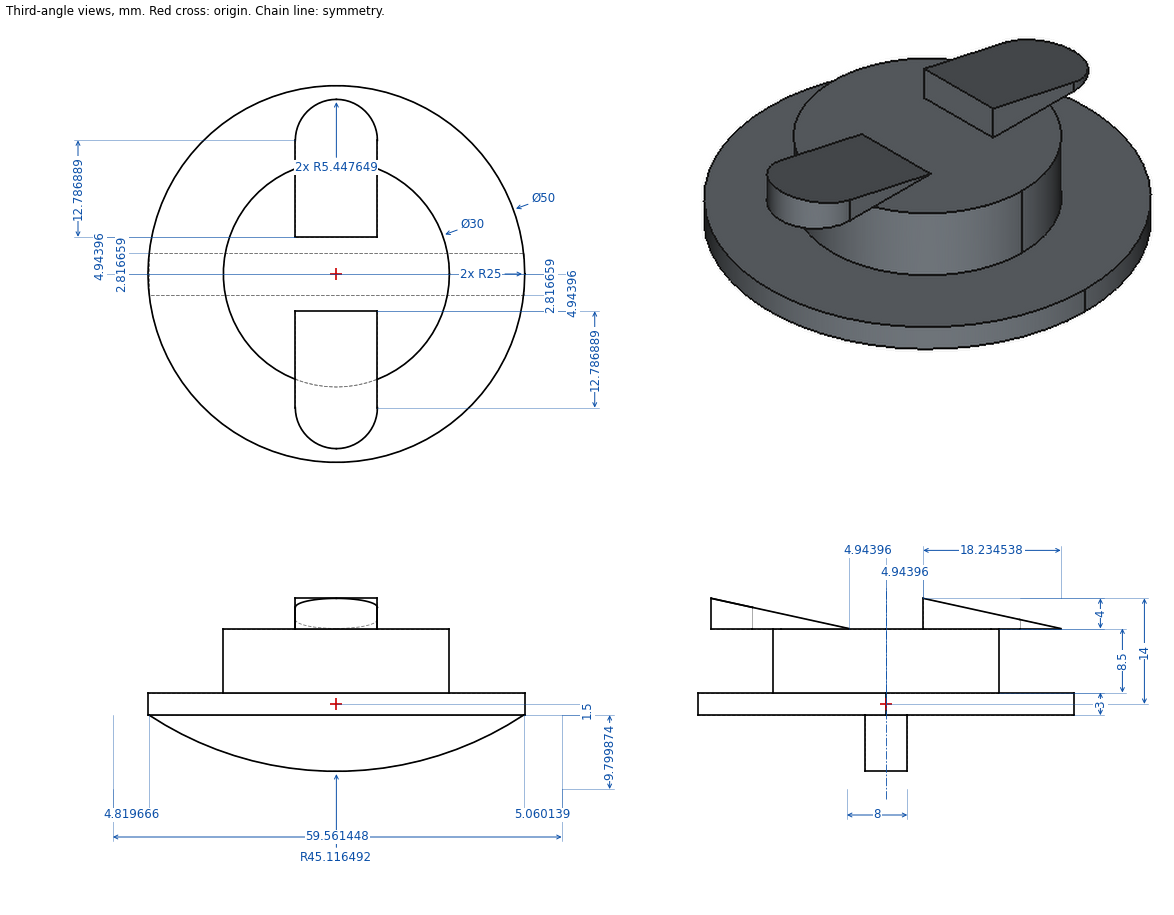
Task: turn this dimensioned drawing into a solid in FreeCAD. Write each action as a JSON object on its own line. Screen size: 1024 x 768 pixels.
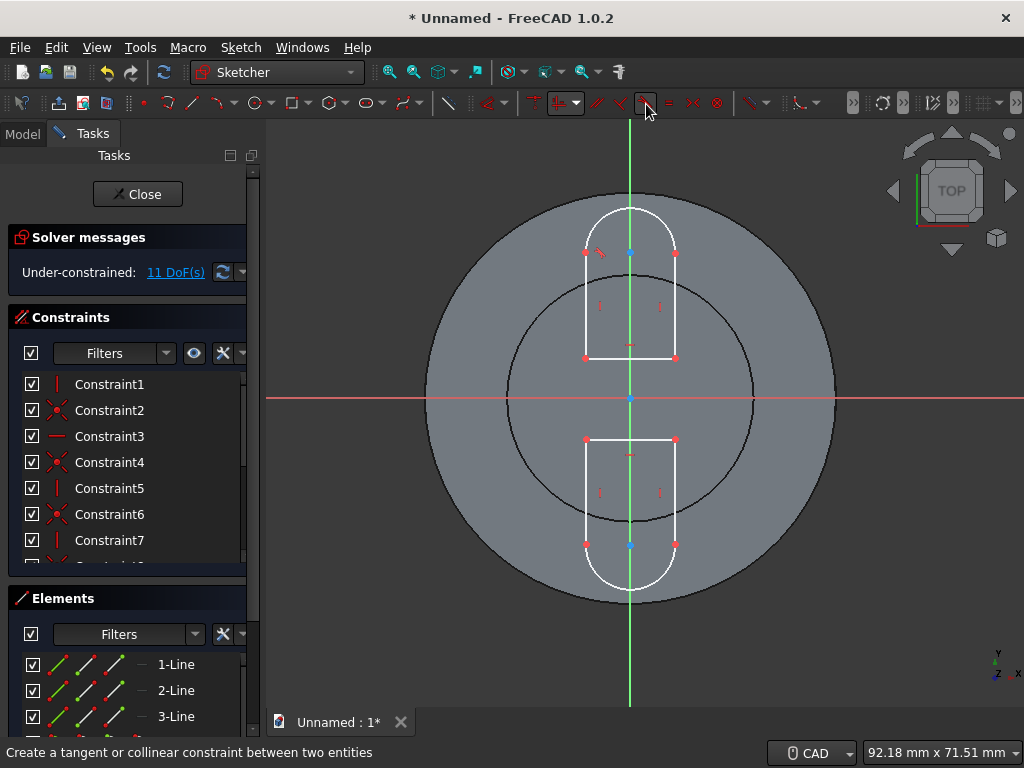
{"action": "left_click", "coordinate": [675, 327]}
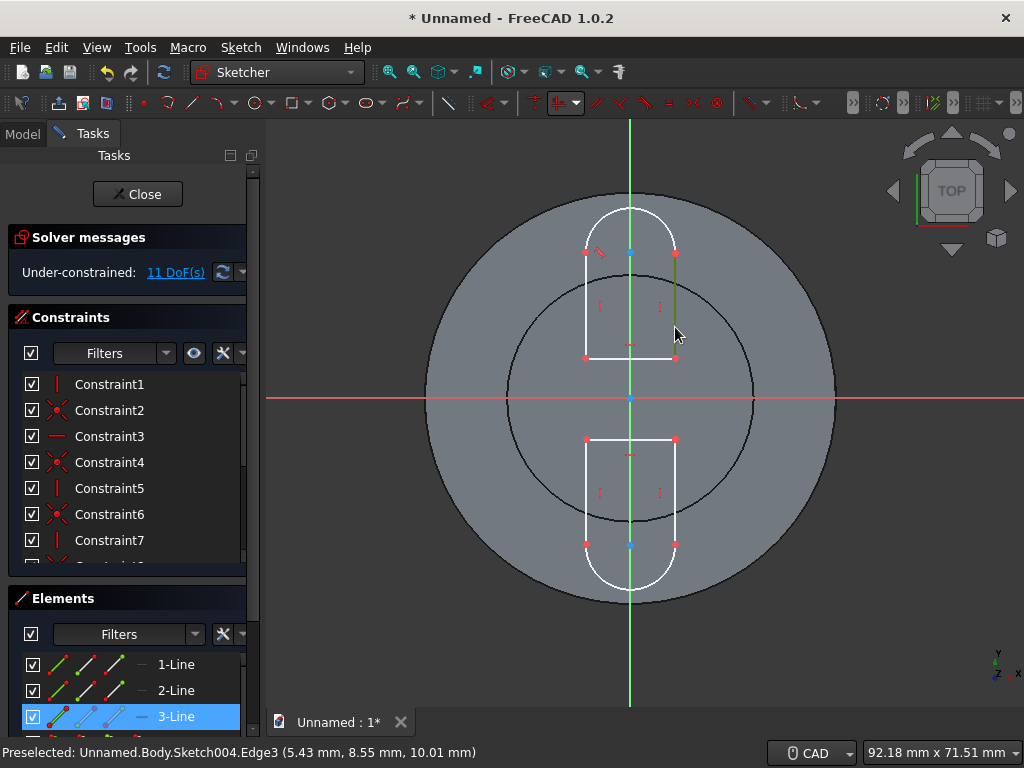
{"action": "left_click", "coordinate": [657, 217]}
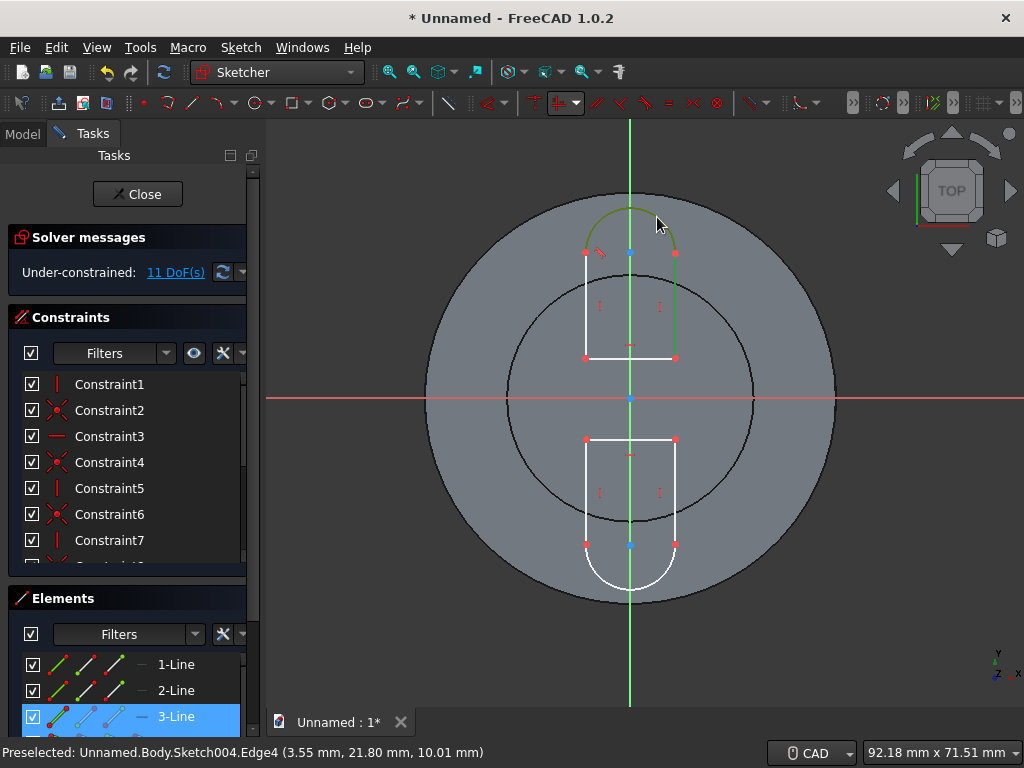
{"action": "left_click", "coordinate": [646, 104]}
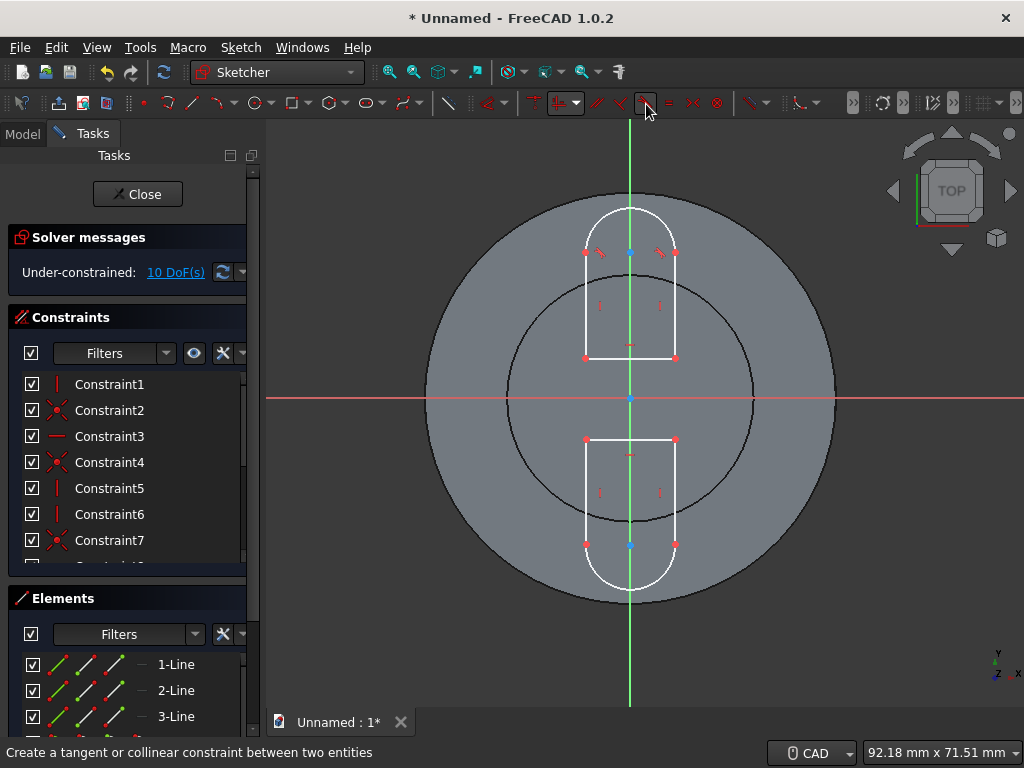
{"action": "left_click", "coordinate": [675, 514]}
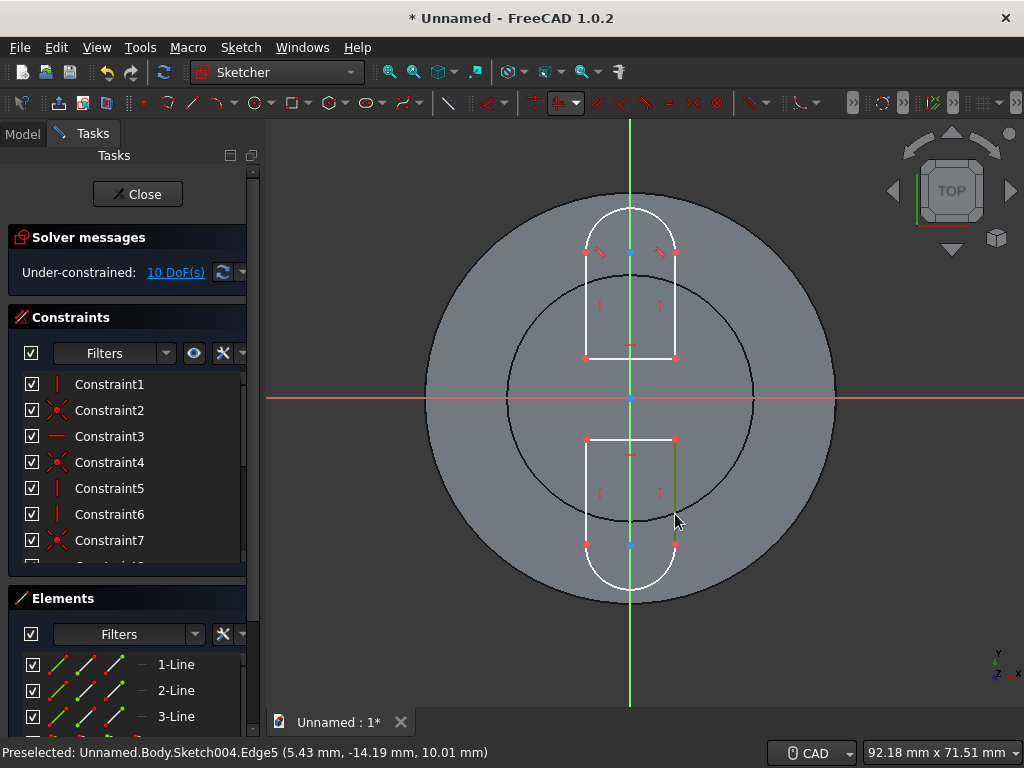
{"action": "left_click", "coordinate": [604, 581]}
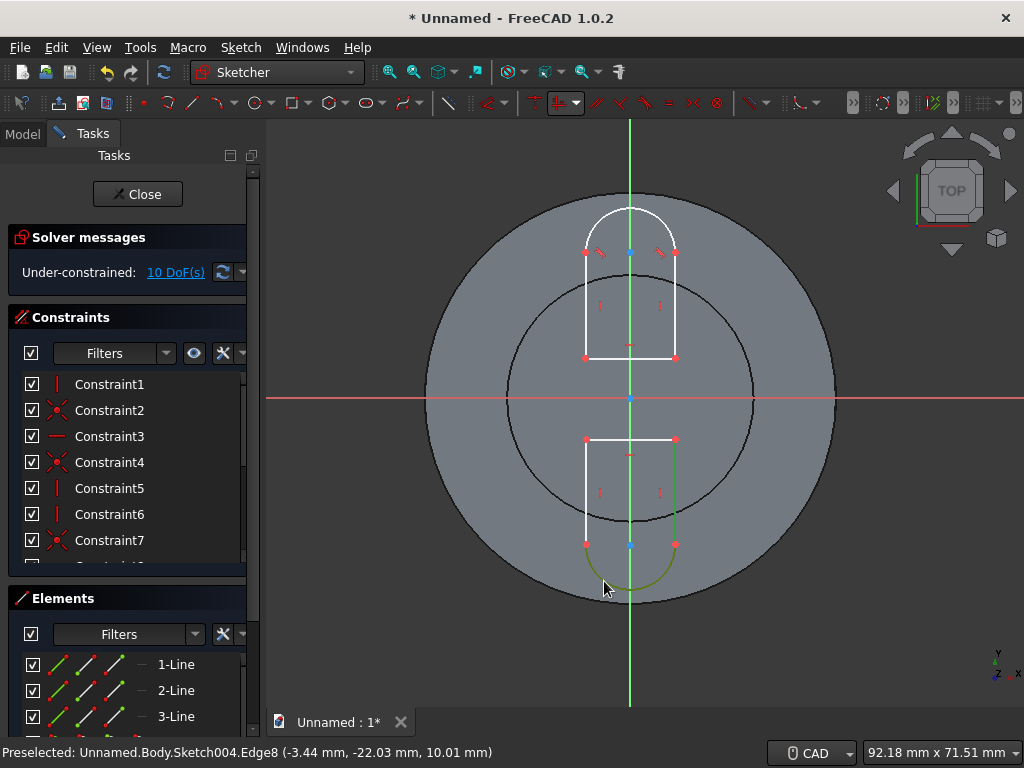
{"action": "left_click", "coordinate": [646, 104]}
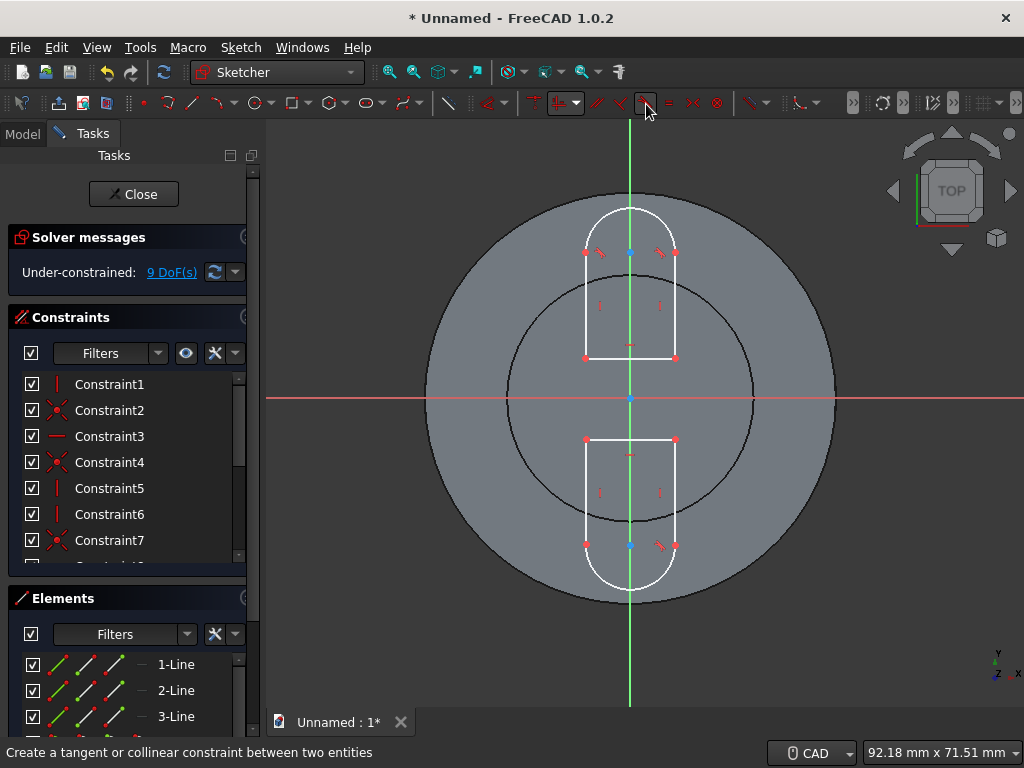
{"action": "left_click", "coordinate": [586, 472]}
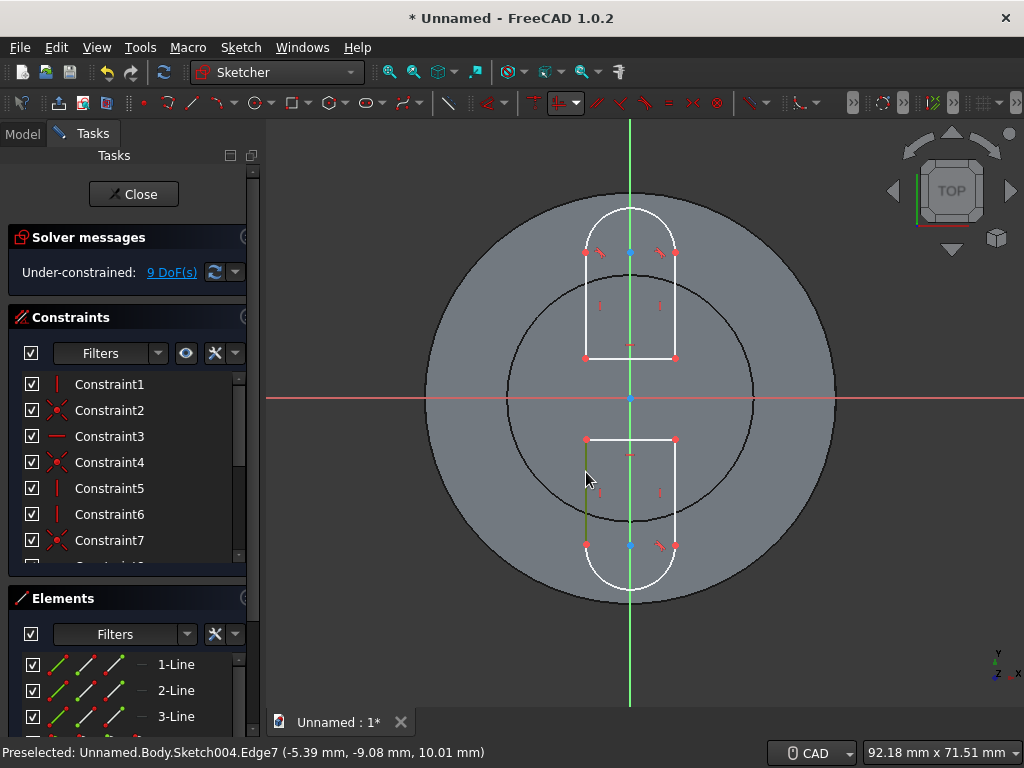
{"action": "left_click", "coordinate": [604, 581]}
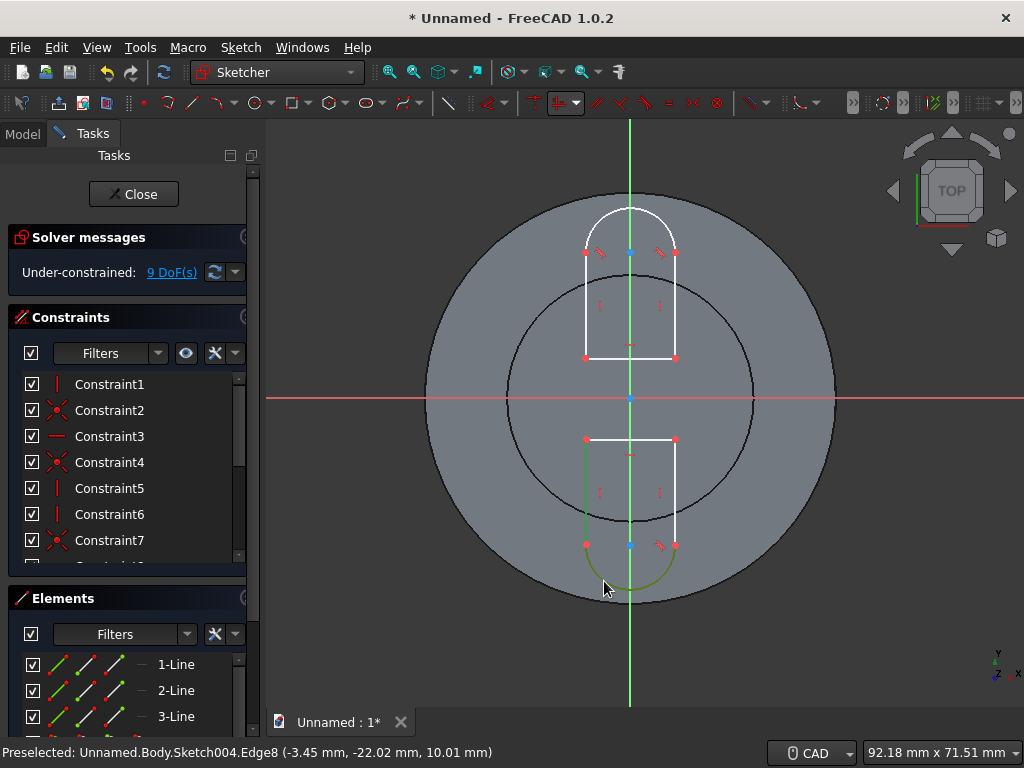
{"action": "left_click", "coordinate": [646, 104]}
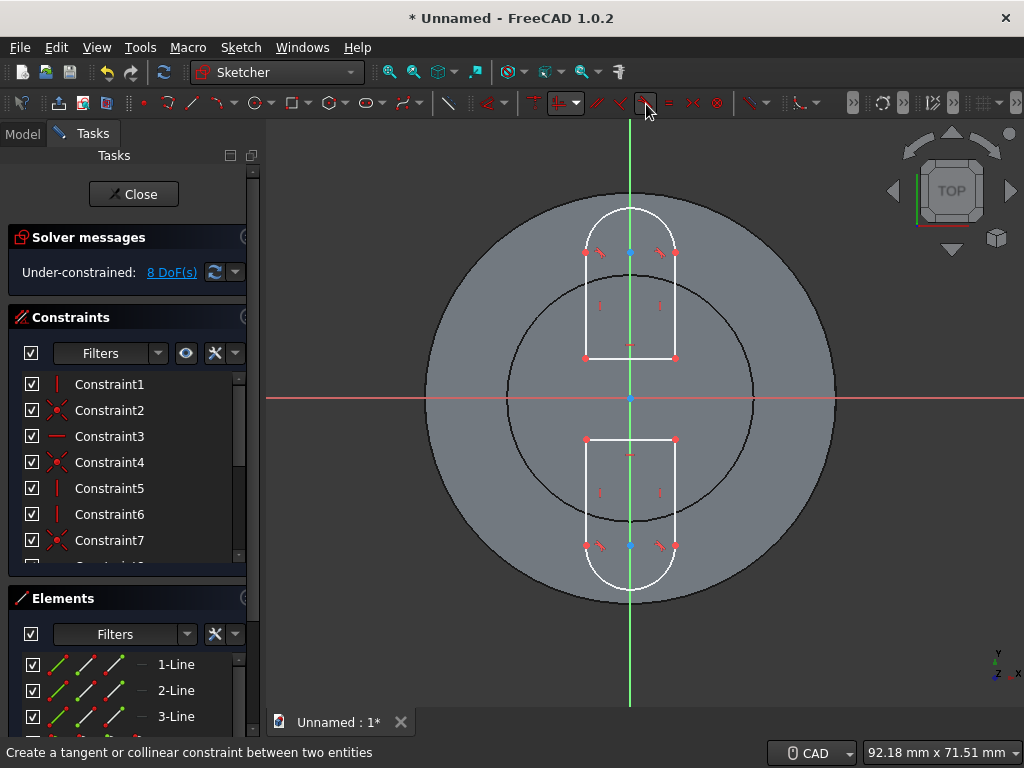
{"action": "left_click", "coordinate": [657, 217]}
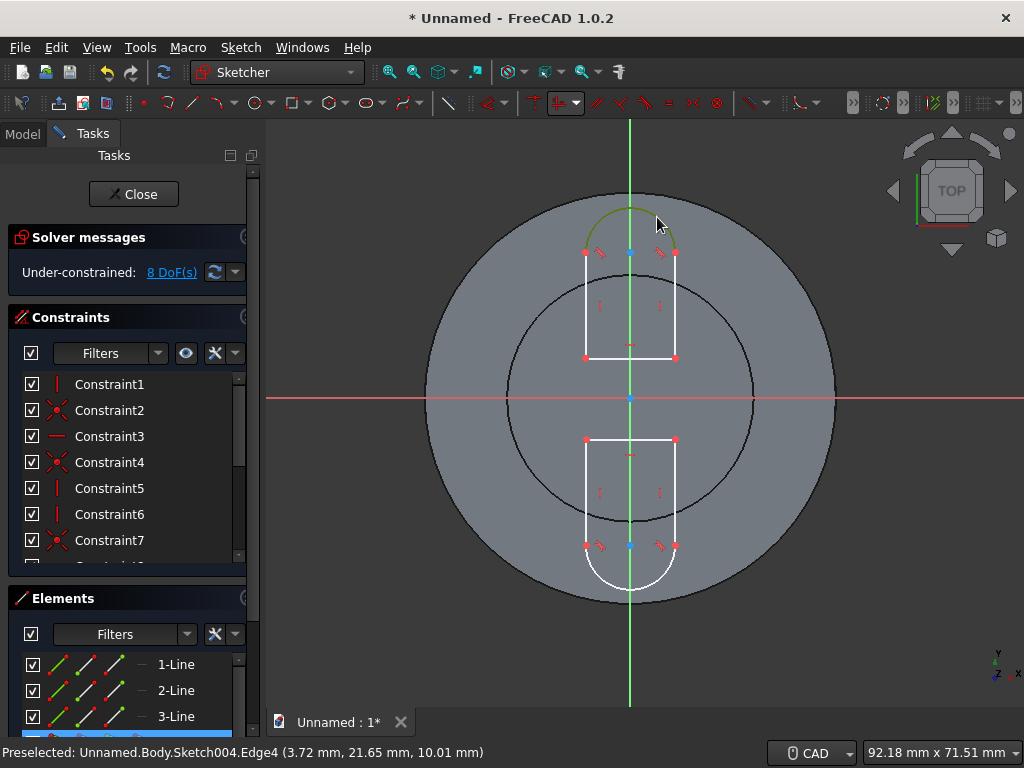
{"action": "left_click", "coordinate": [604, 581]}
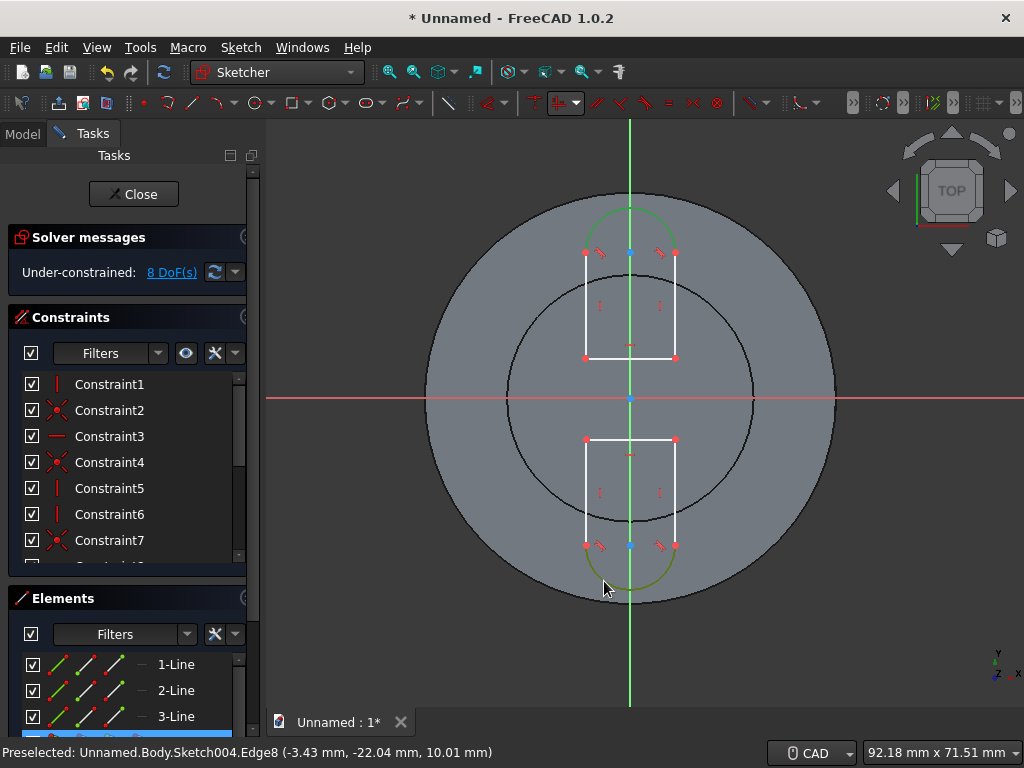
{"action": "left_click", "coordinate": [670, 104]}